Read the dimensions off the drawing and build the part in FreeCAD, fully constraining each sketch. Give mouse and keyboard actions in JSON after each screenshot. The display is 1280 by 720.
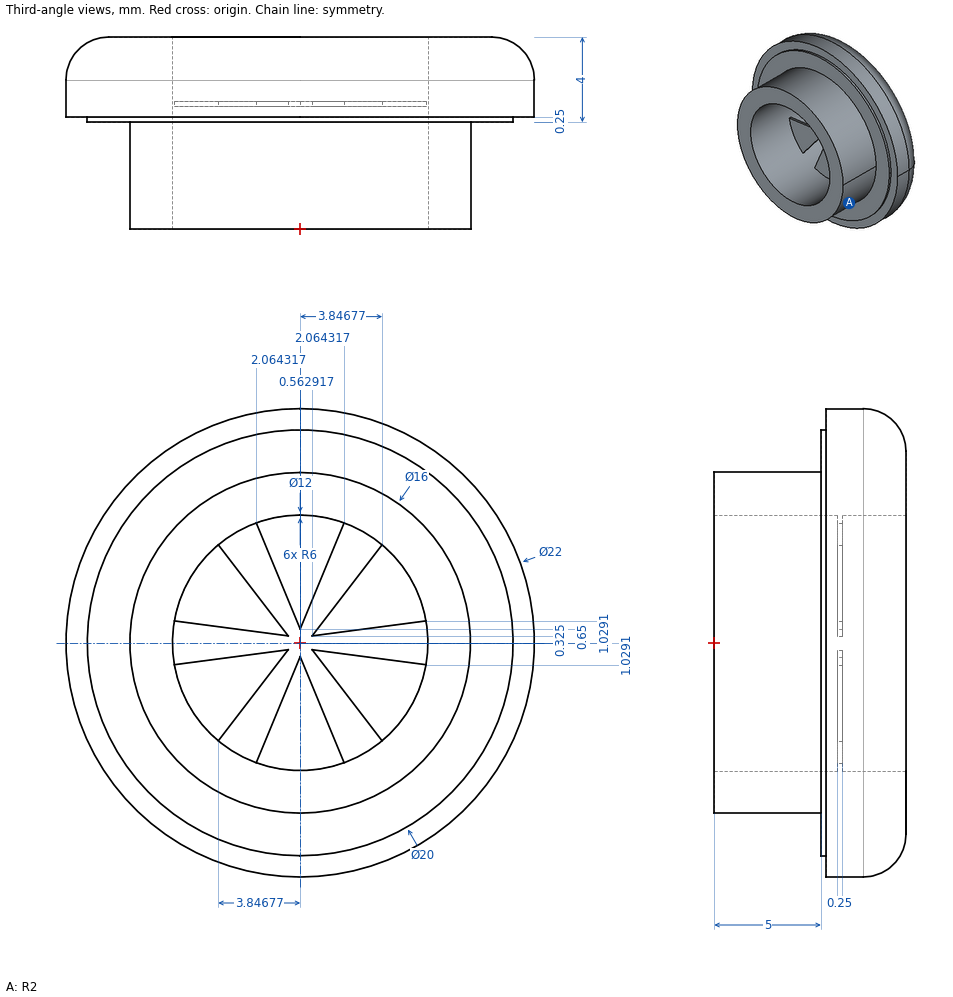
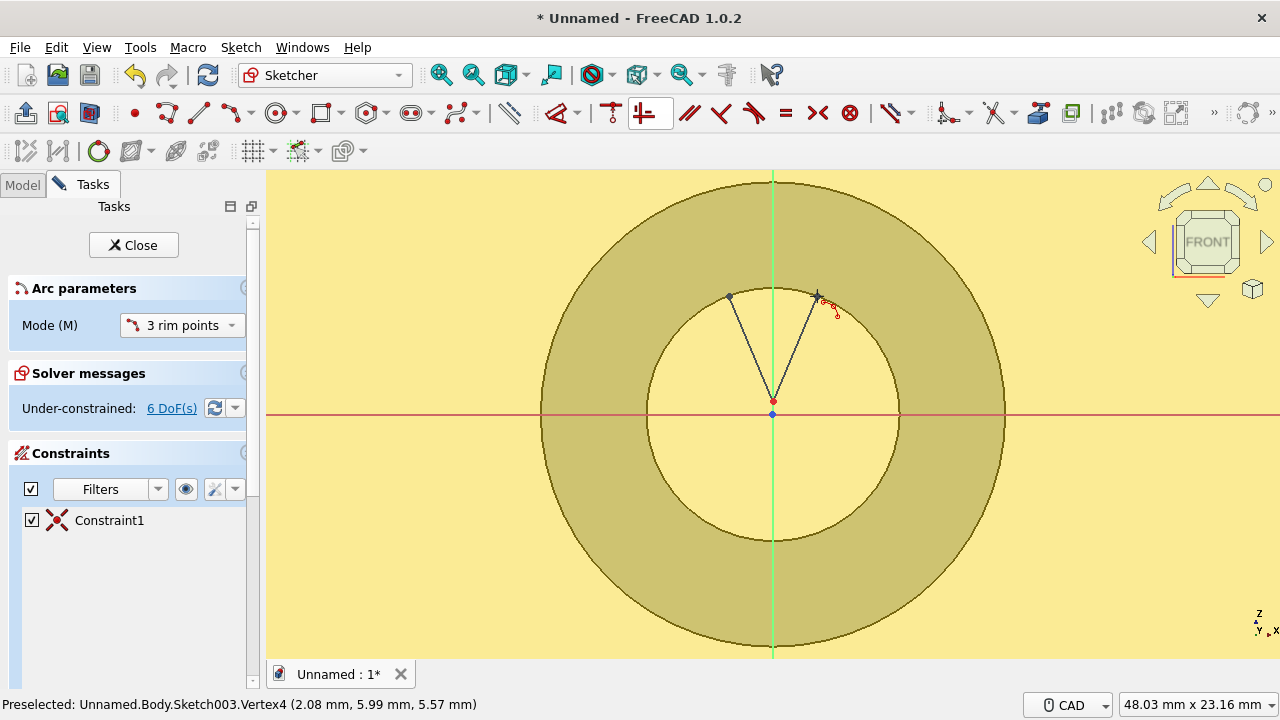
{"action": "left_click", "coordinate": [817, 297]}
{"action": "left_click", "coordinate": [729, 297]}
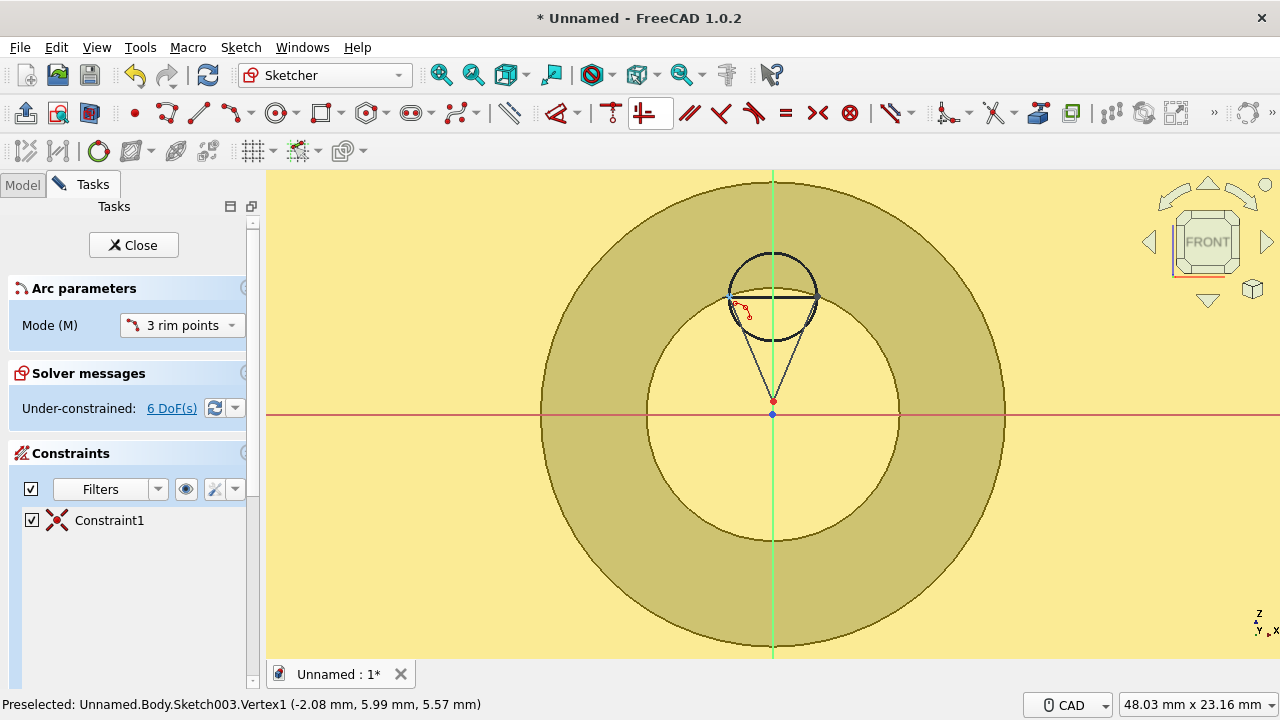
{"action": "scroll", "coordinate": [782, 288], "scroll_direction": "up", "scroll_amount": 4}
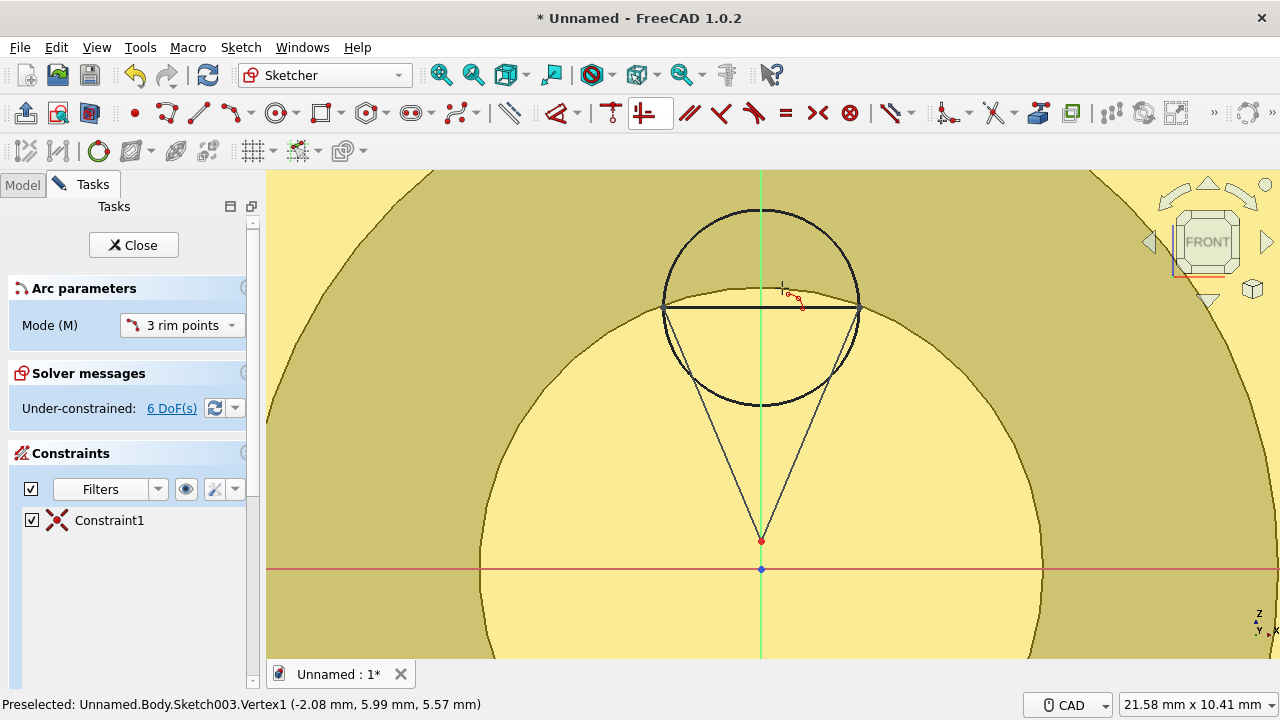
{"action": "left_click", "coordinate": [781, 288]}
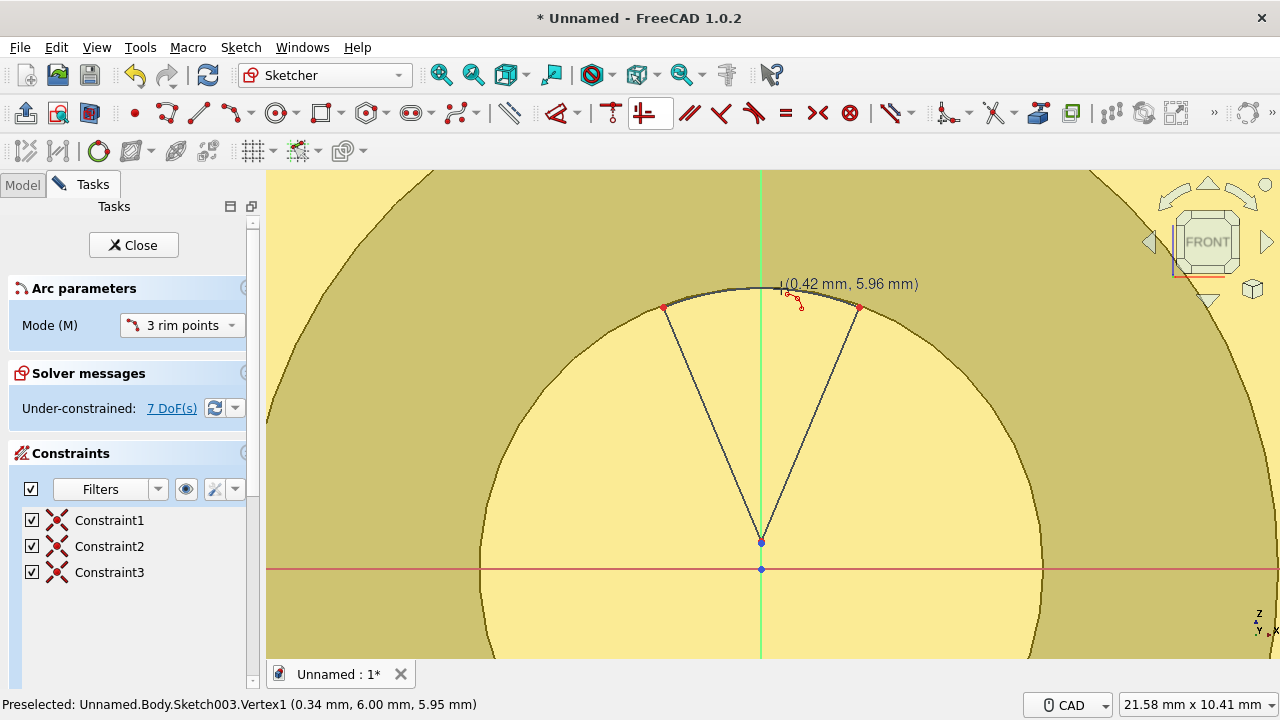
{"action": "key", "text": "g m"}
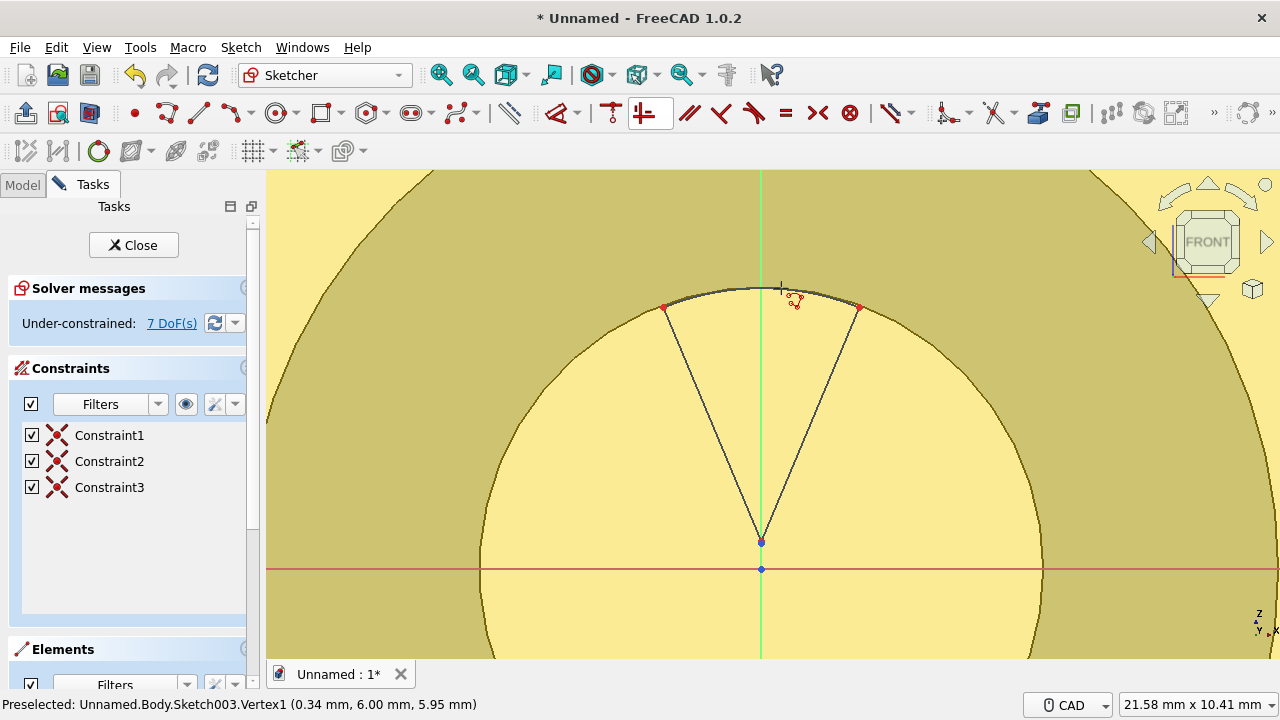
{"action": "left_click", "coordinate": [942, 353]}
{"action": "left_click", "coordinate": [788, 554]}
{"action": "left_click", "coordinate": [1039, 521]}
{"action": "right_click", "coordinate": [1039, 521]}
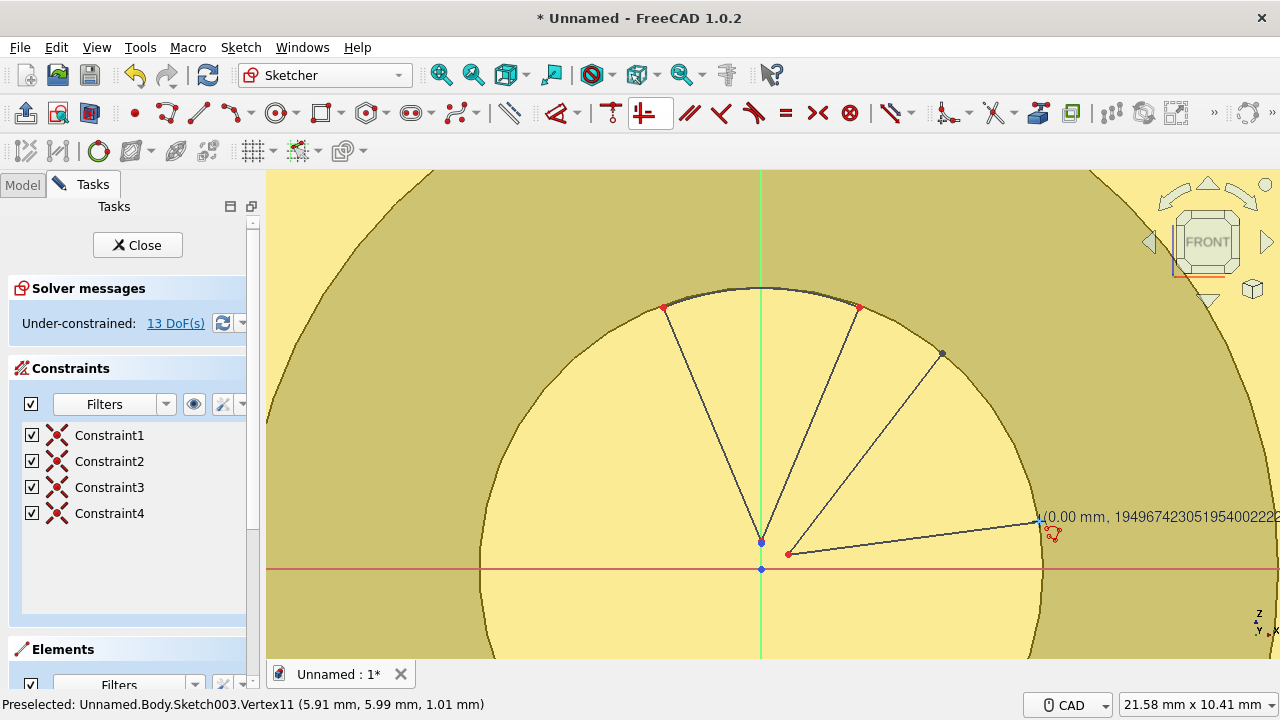
{"action": "key", "text": "g 3 a"}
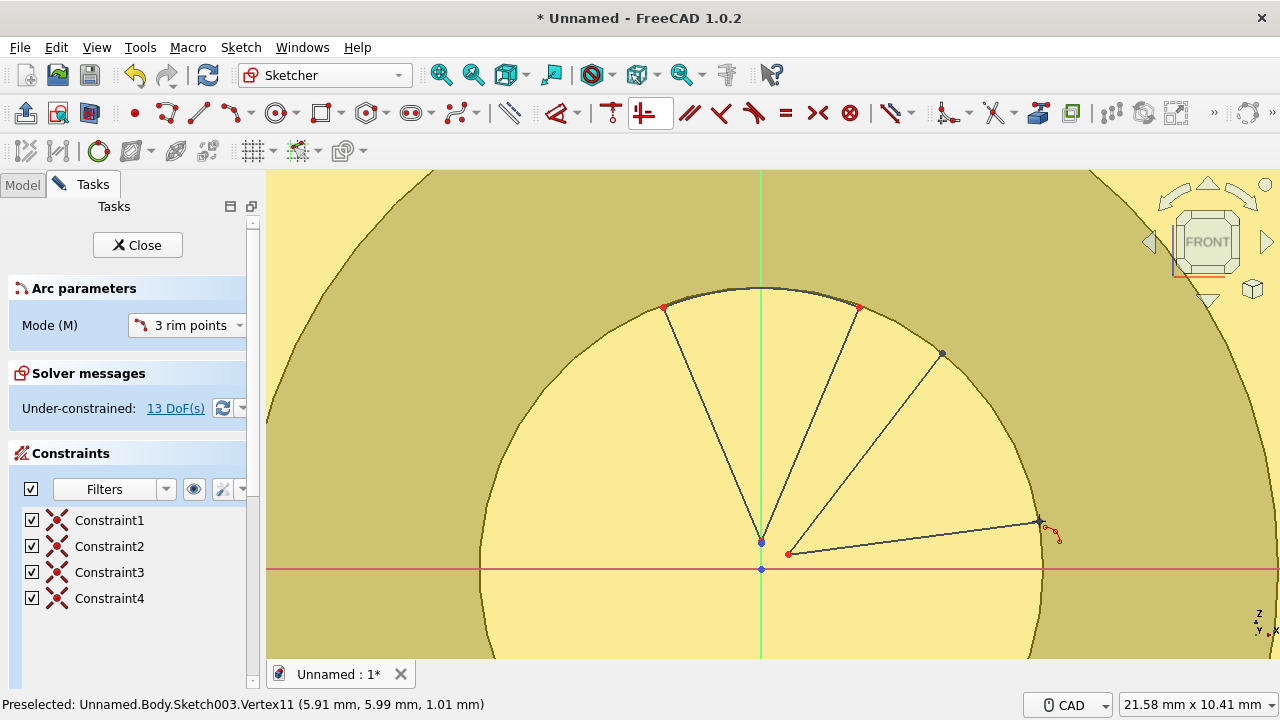
{"action": "left_click", "coordinate": [1039, 522]}
{"action": "left_click", "coordinate": [942, 354]}
{"action": "left_click", "coordinate": [1005, 428]}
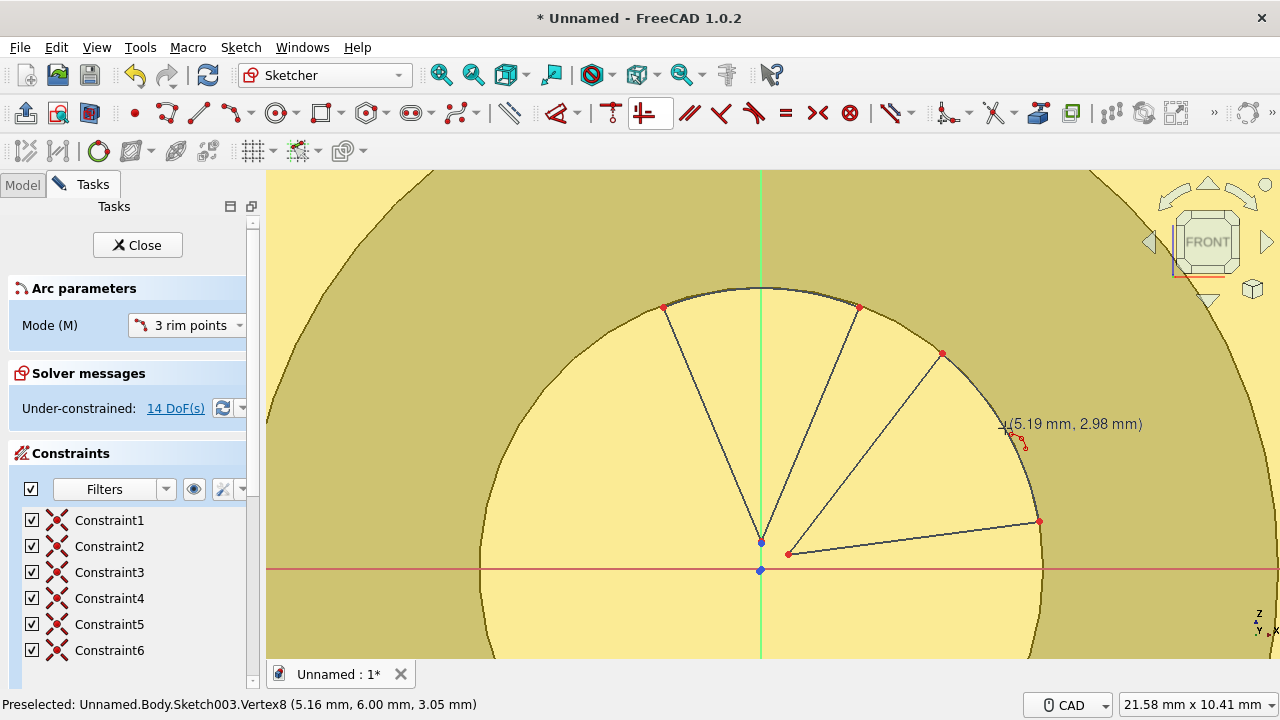
{"action": "left_click", "coordinate": [168, 114]}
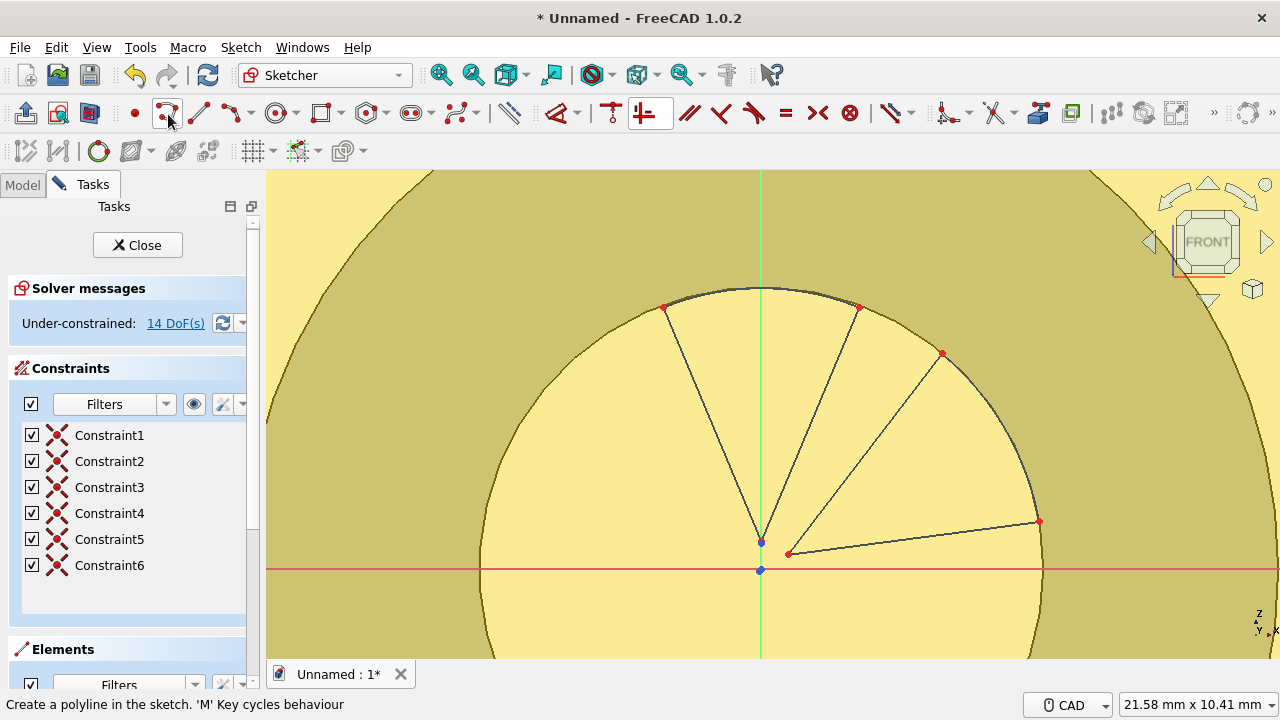
{"action": "left_click", "coordinate": [1039, 618]}
{"action": "left_click", "coordinate": [788, 585]}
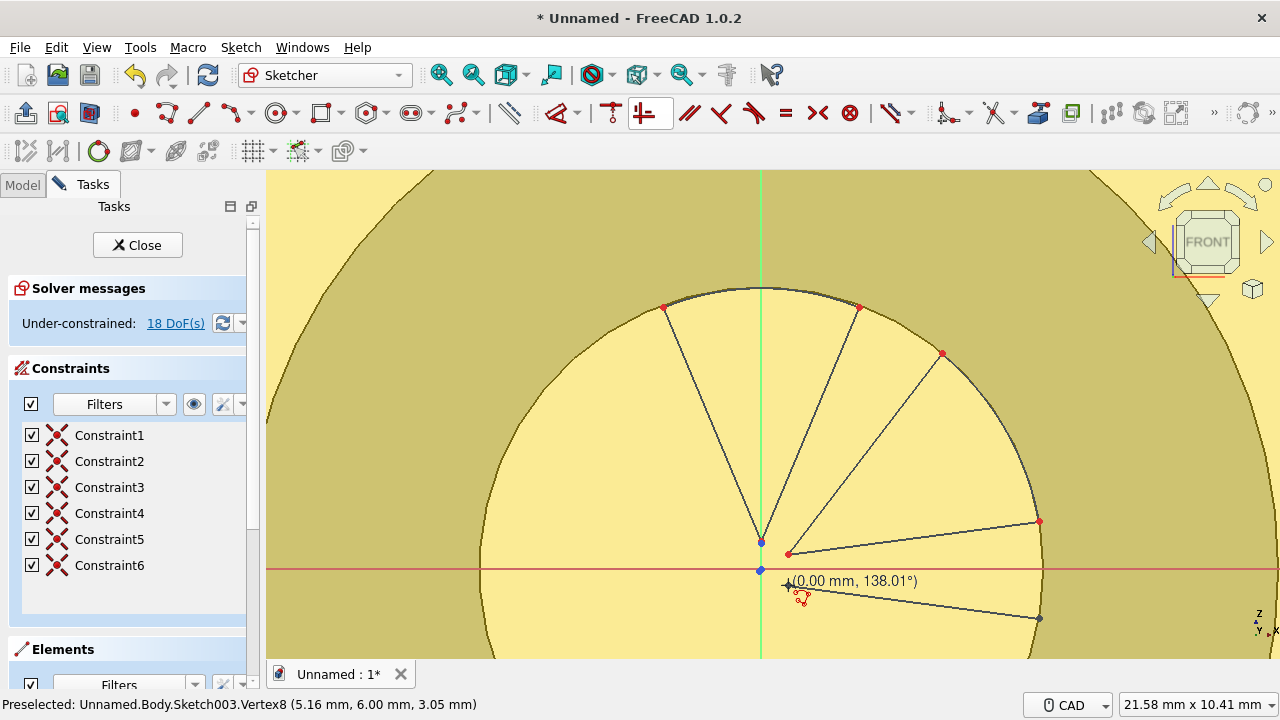
{"action": "scroll", "coordinate": [635, 226], "scroll_direction": "down", "scroll_amount": 3}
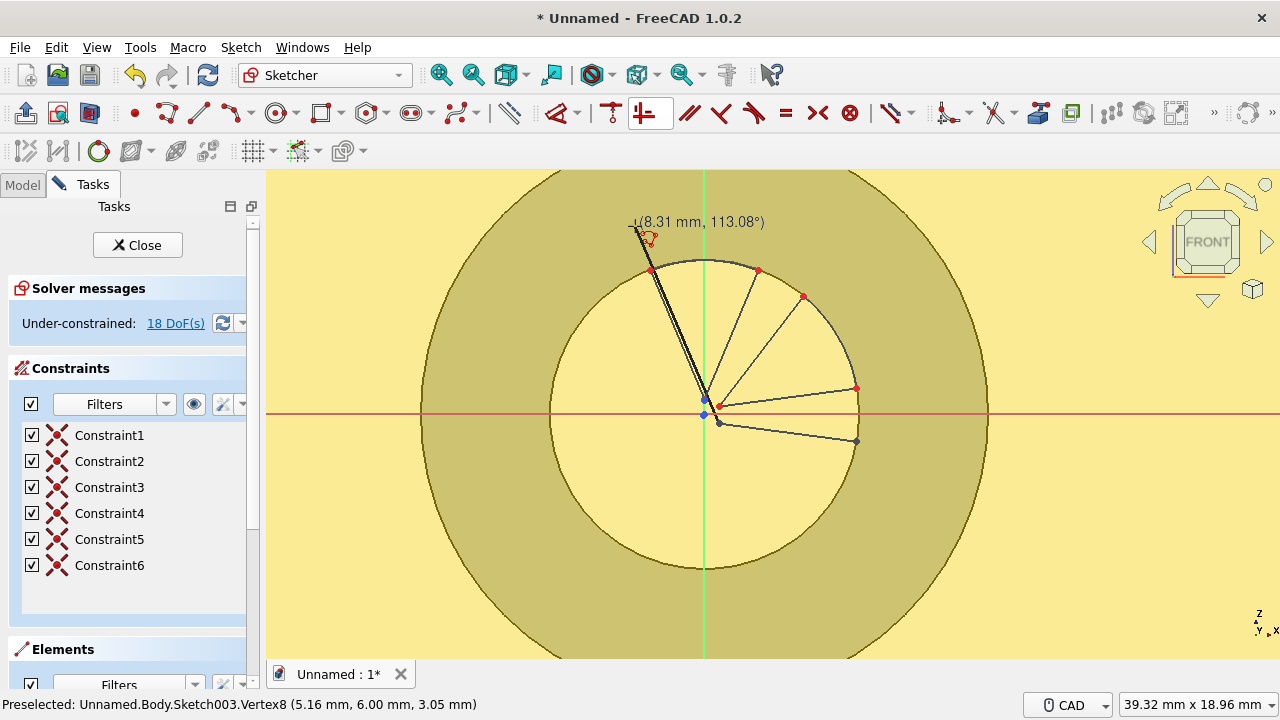
{"action": "left_click", "coordinate": [804, 533]}
{"action": "right_click", "coordinate": [804, 533]}